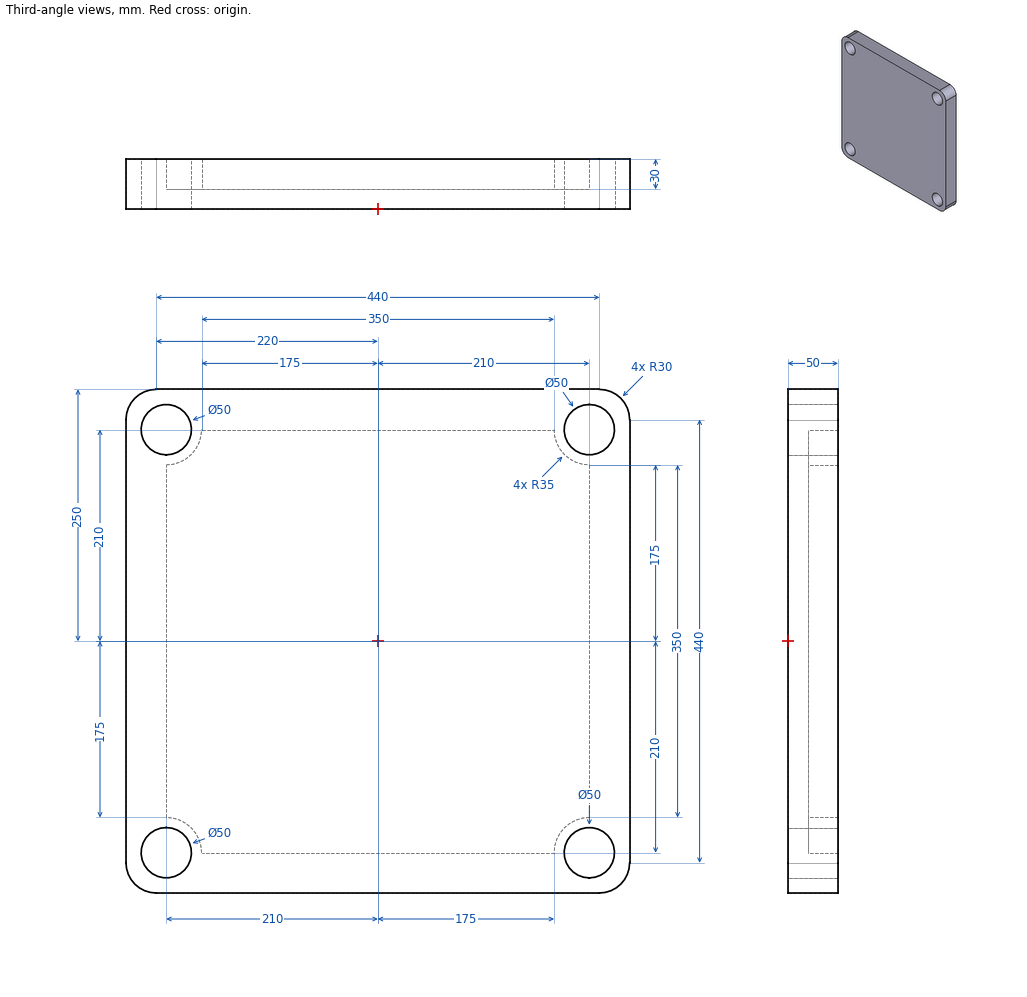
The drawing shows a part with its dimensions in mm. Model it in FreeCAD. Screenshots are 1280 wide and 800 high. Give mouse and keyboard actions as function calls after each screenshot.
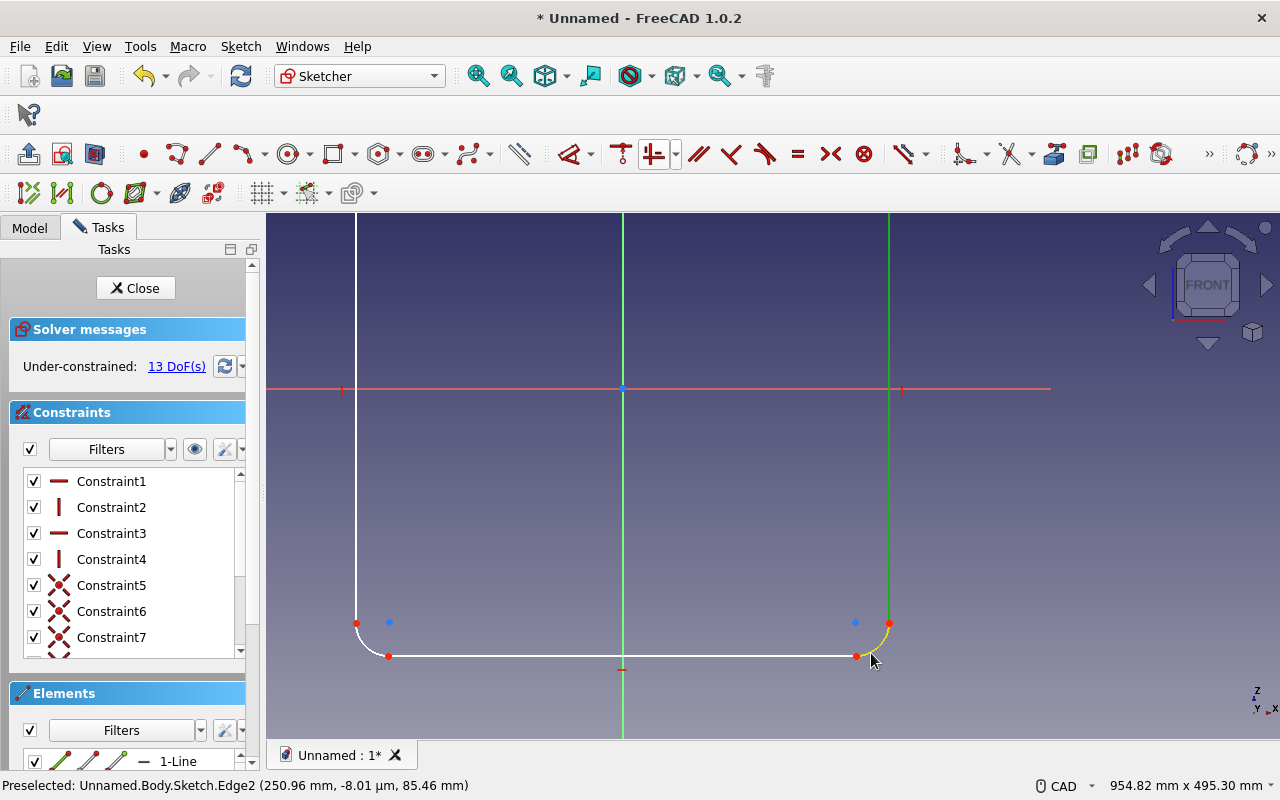
click(871, 652)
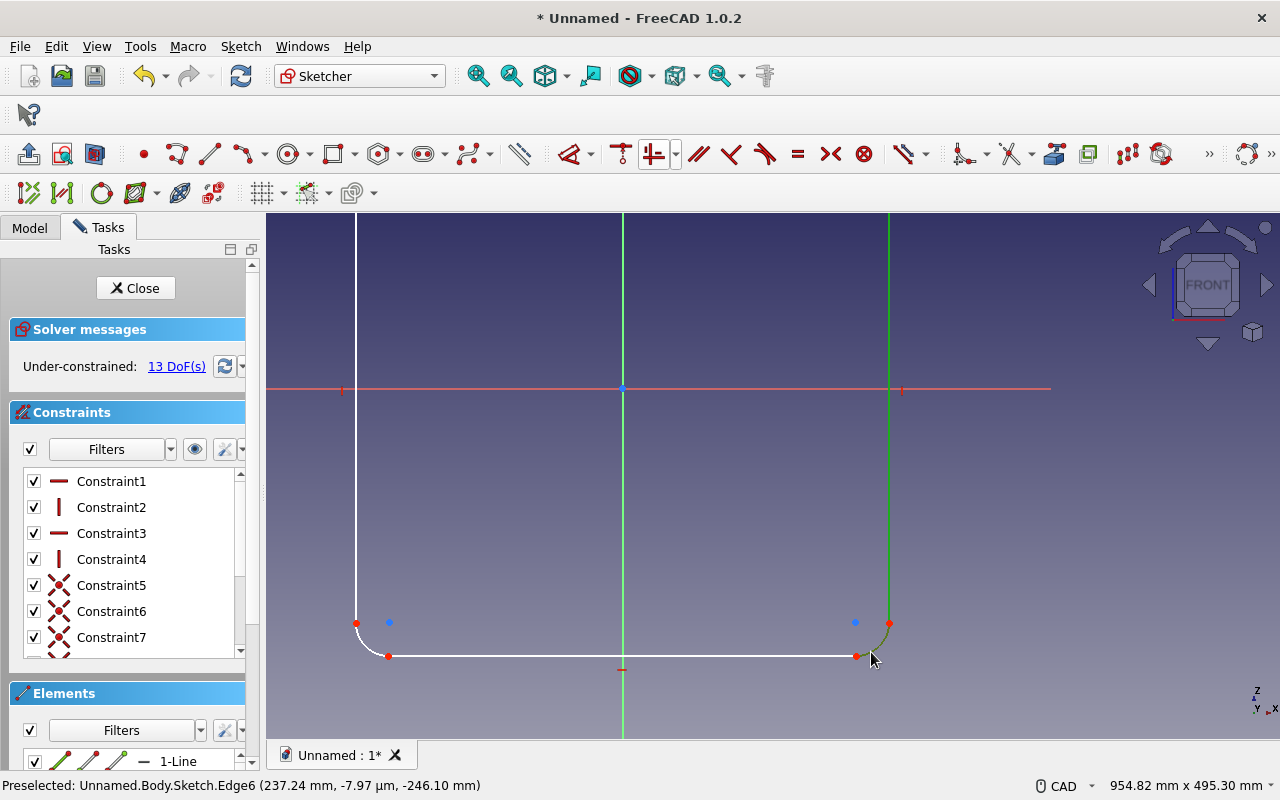
click(765, 154)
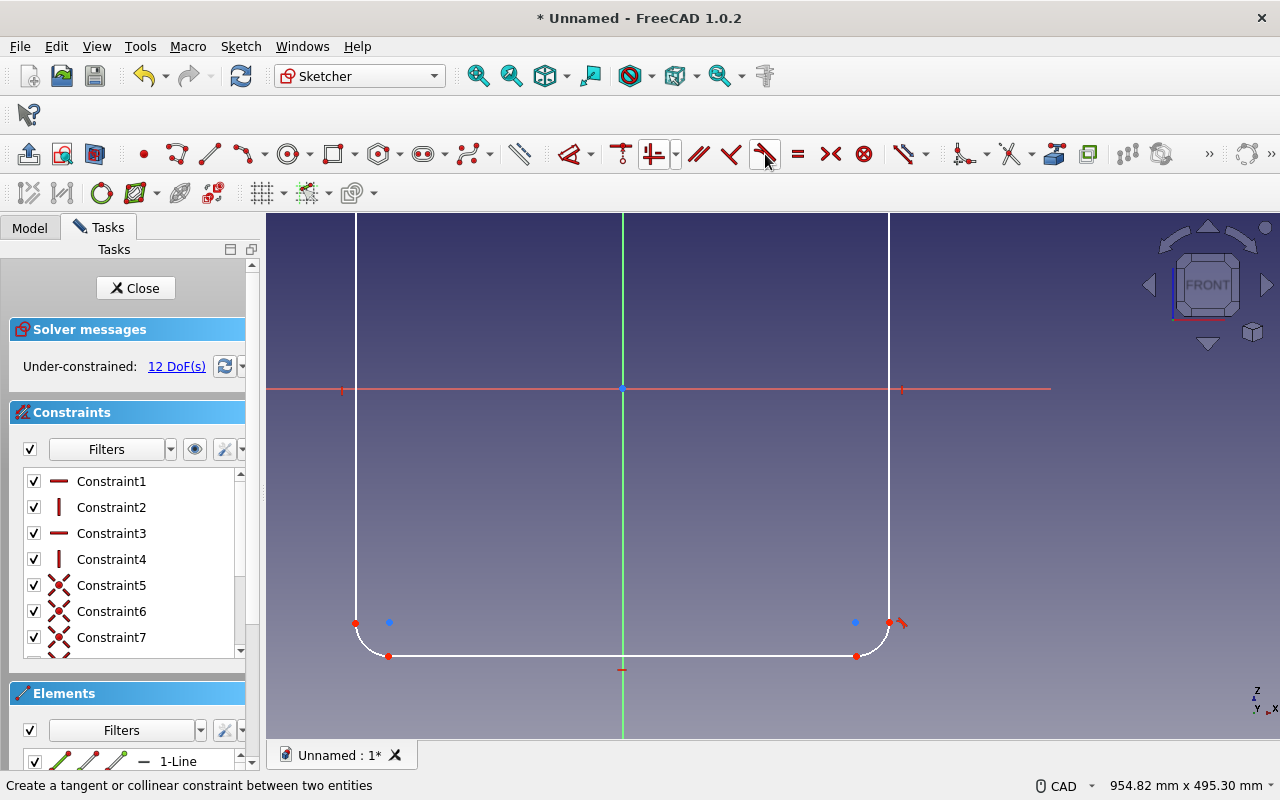
click(716, 656)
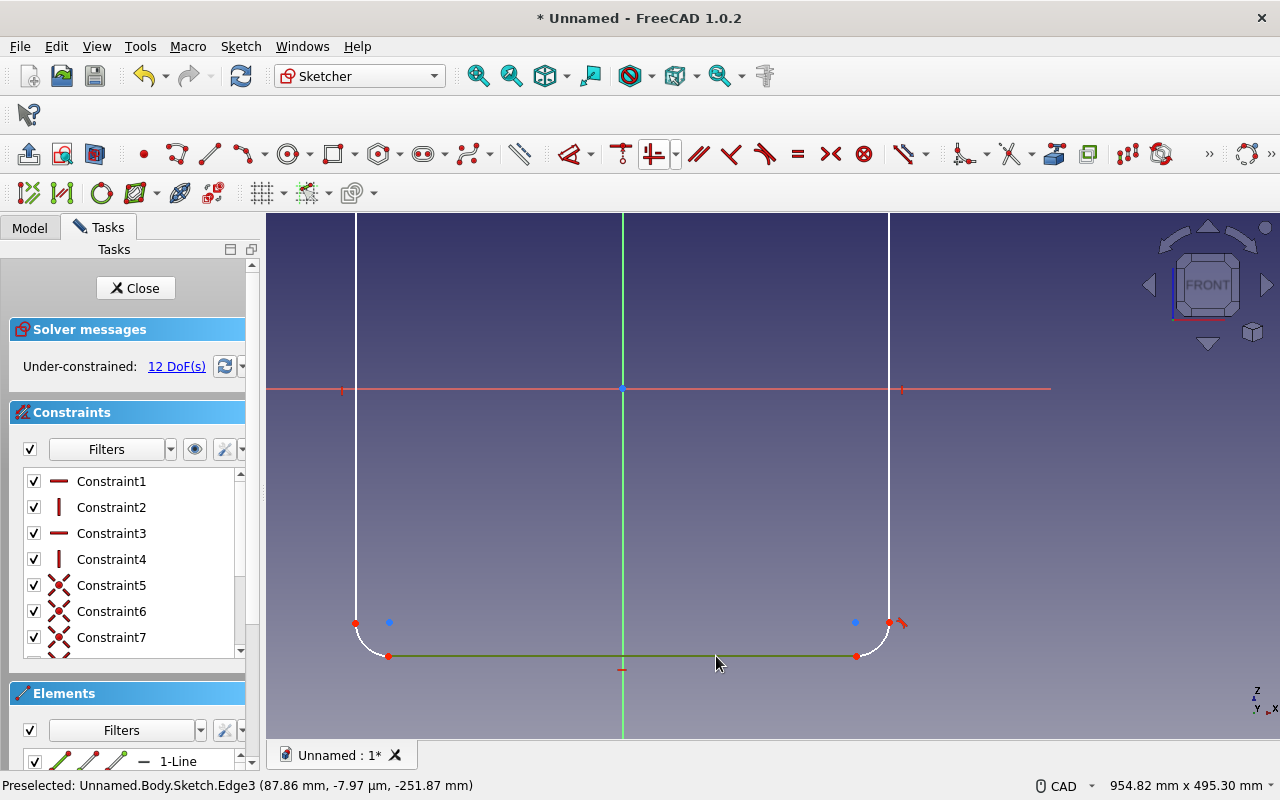
click(872, 652)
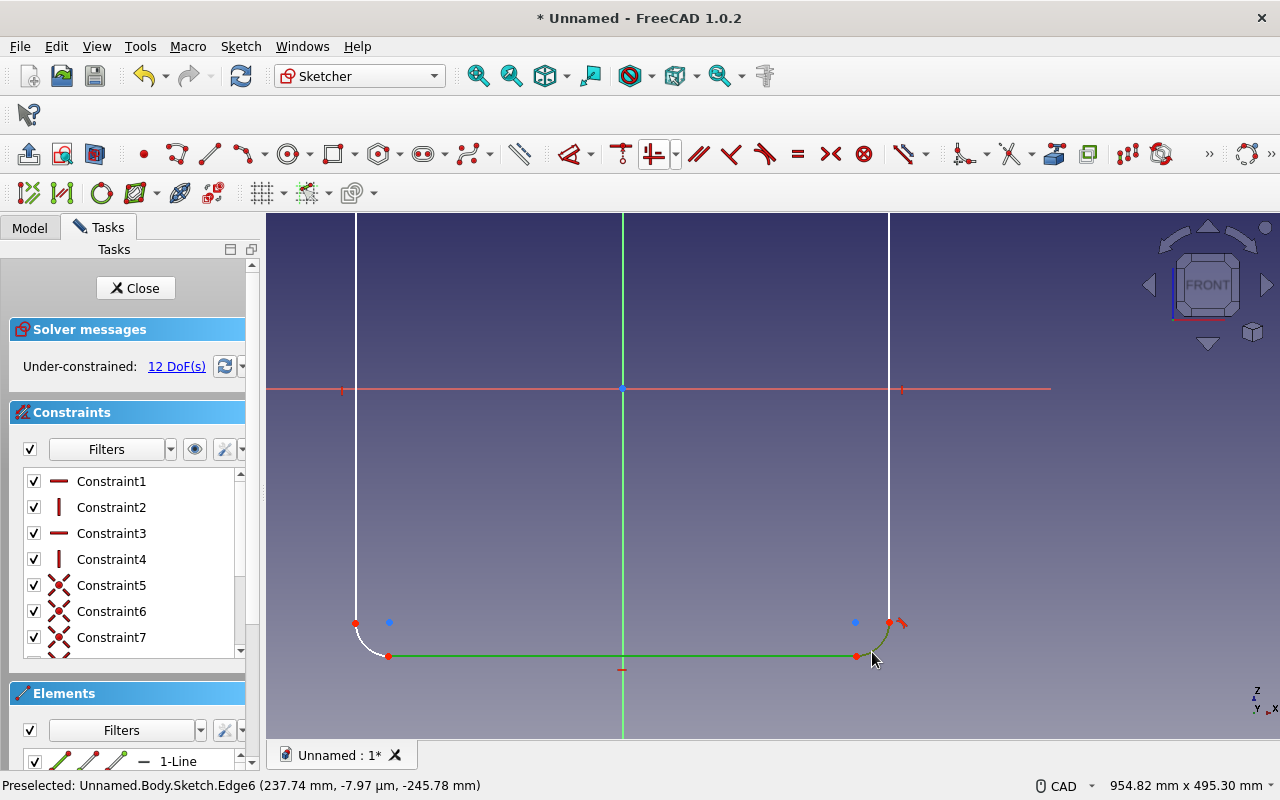
click(765, 154)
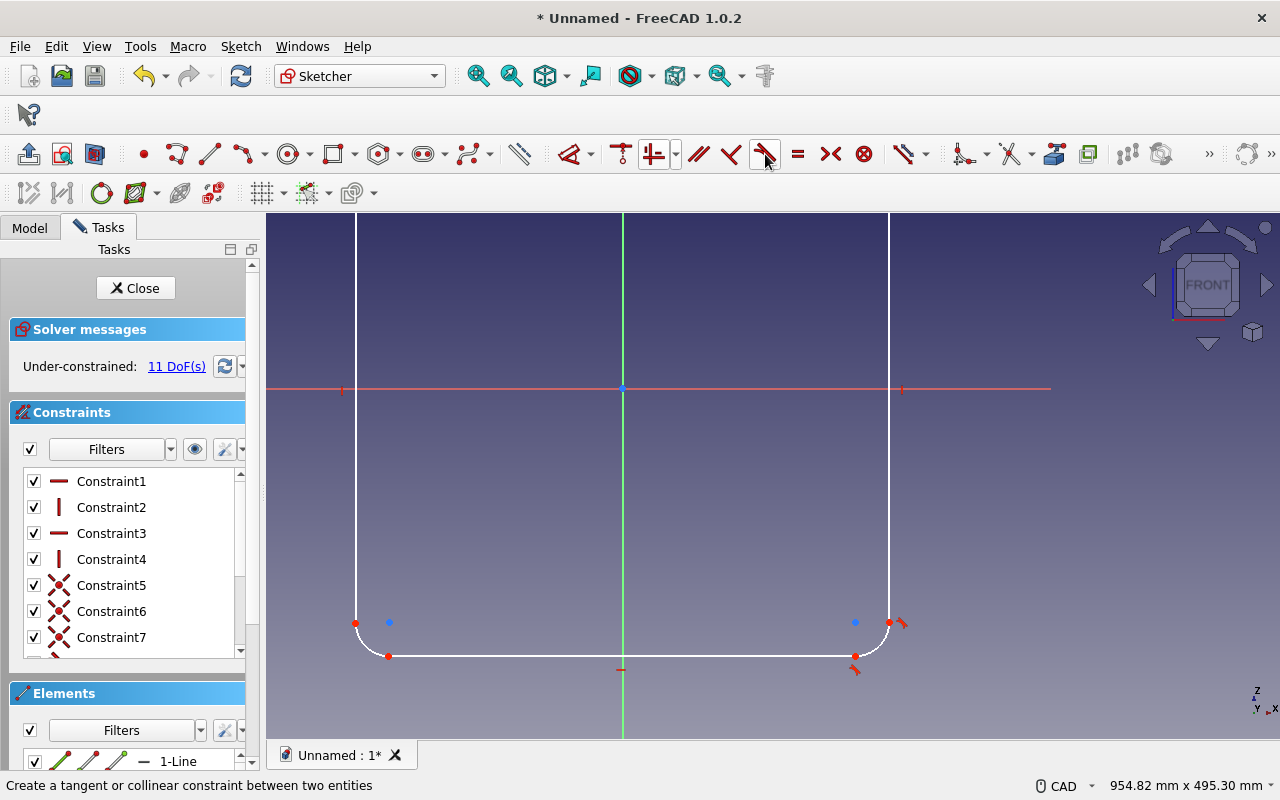
click(715, 656)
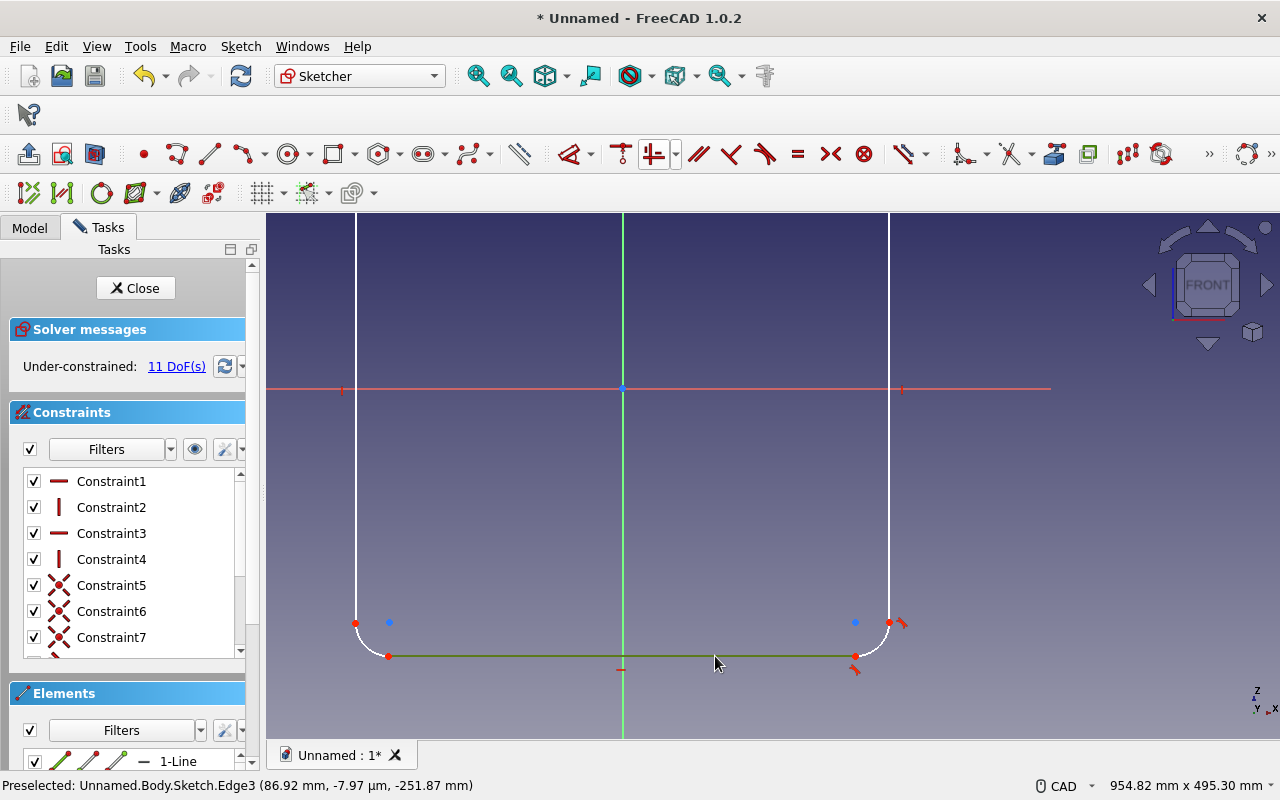
click(360, 638)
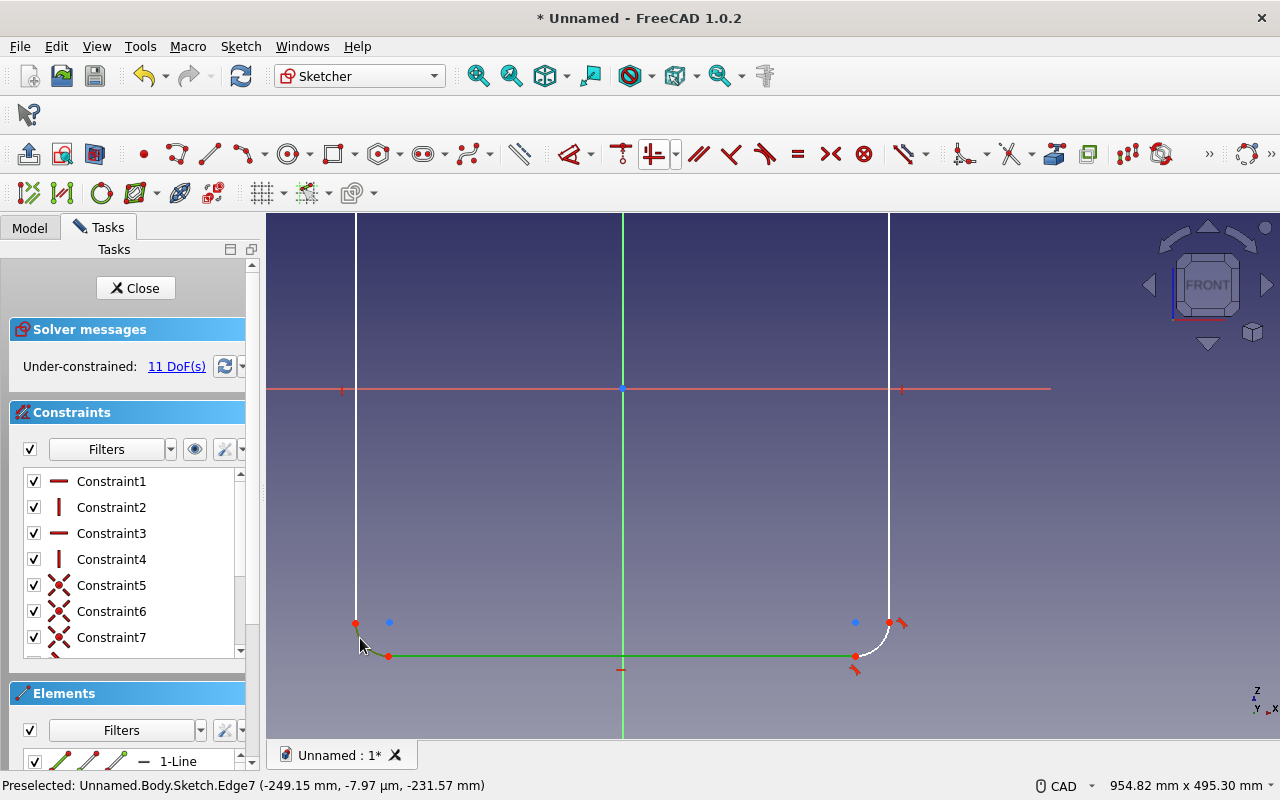
click(765, 154)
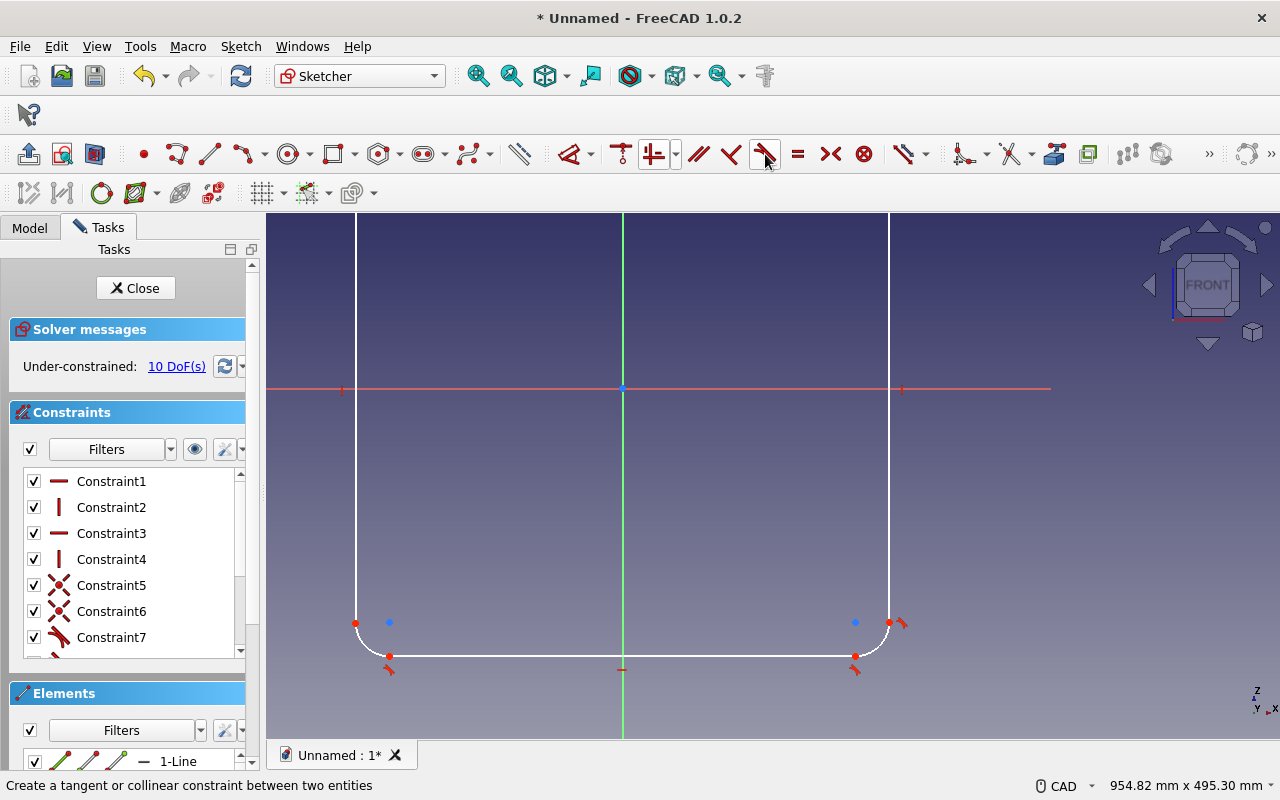
click(356, 484)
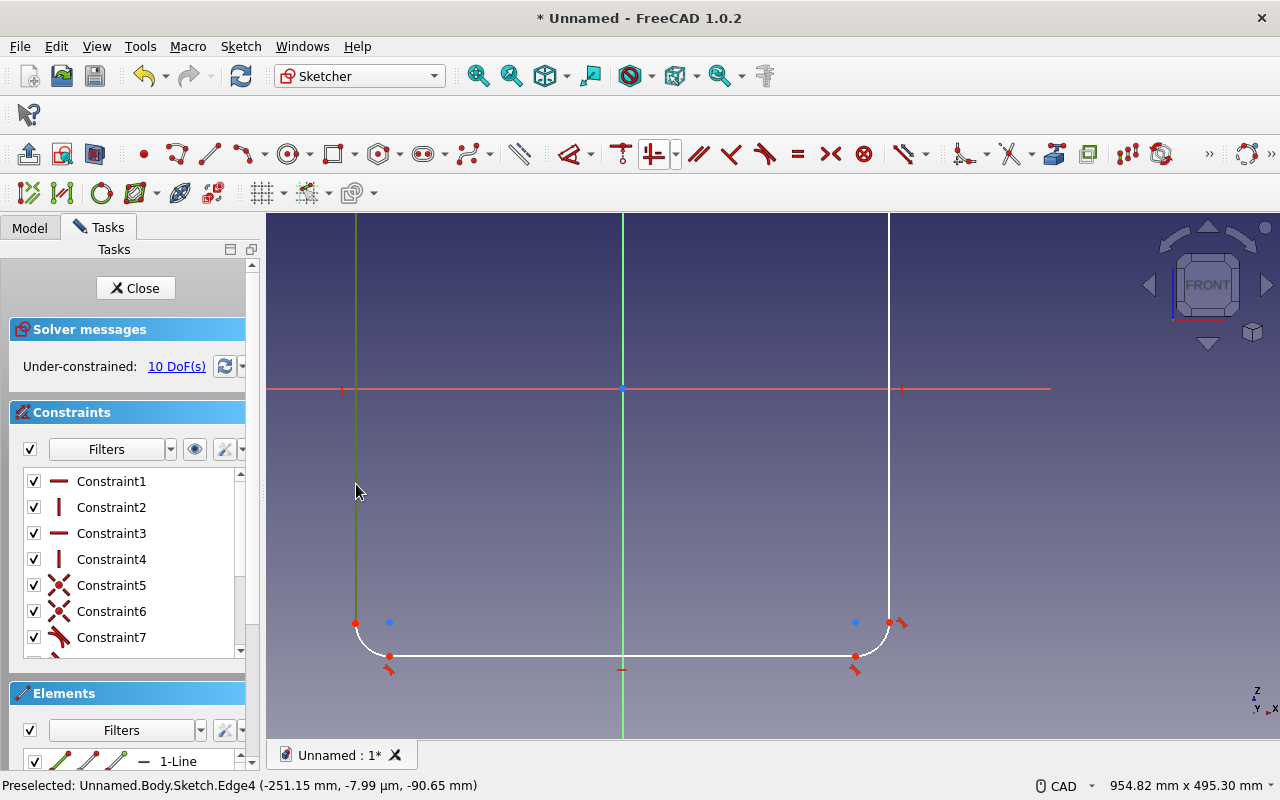
click(360, 639)